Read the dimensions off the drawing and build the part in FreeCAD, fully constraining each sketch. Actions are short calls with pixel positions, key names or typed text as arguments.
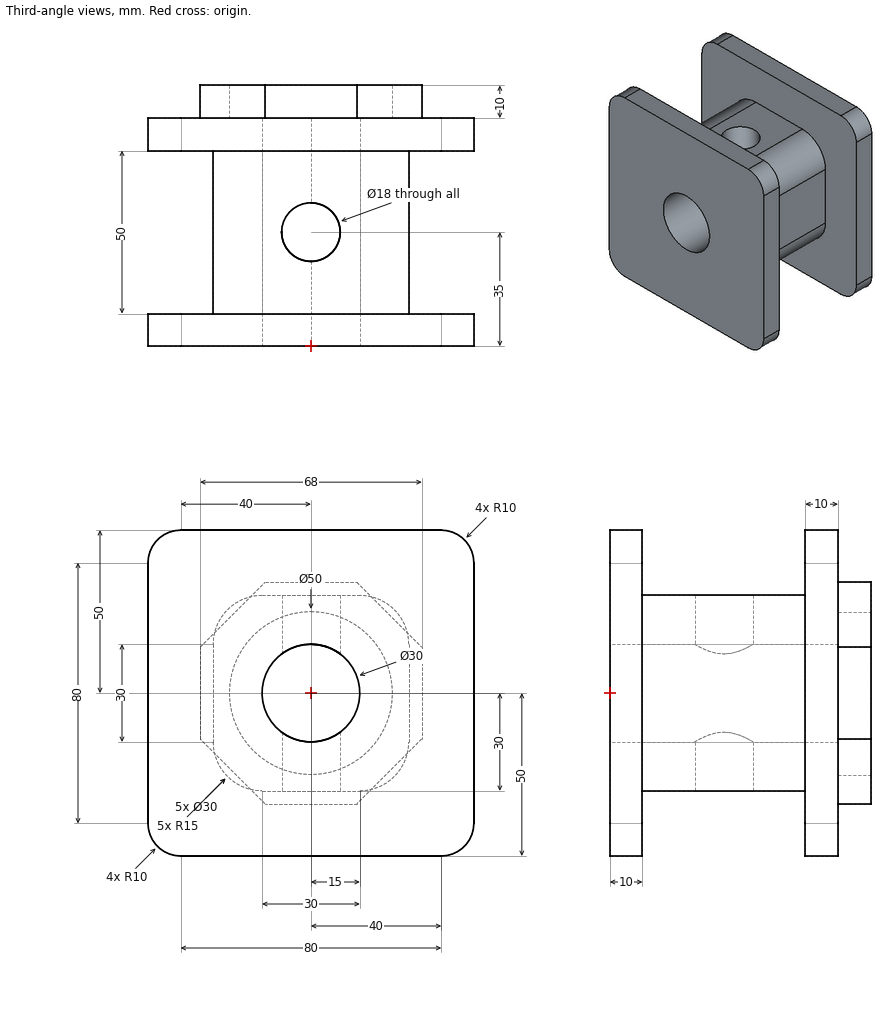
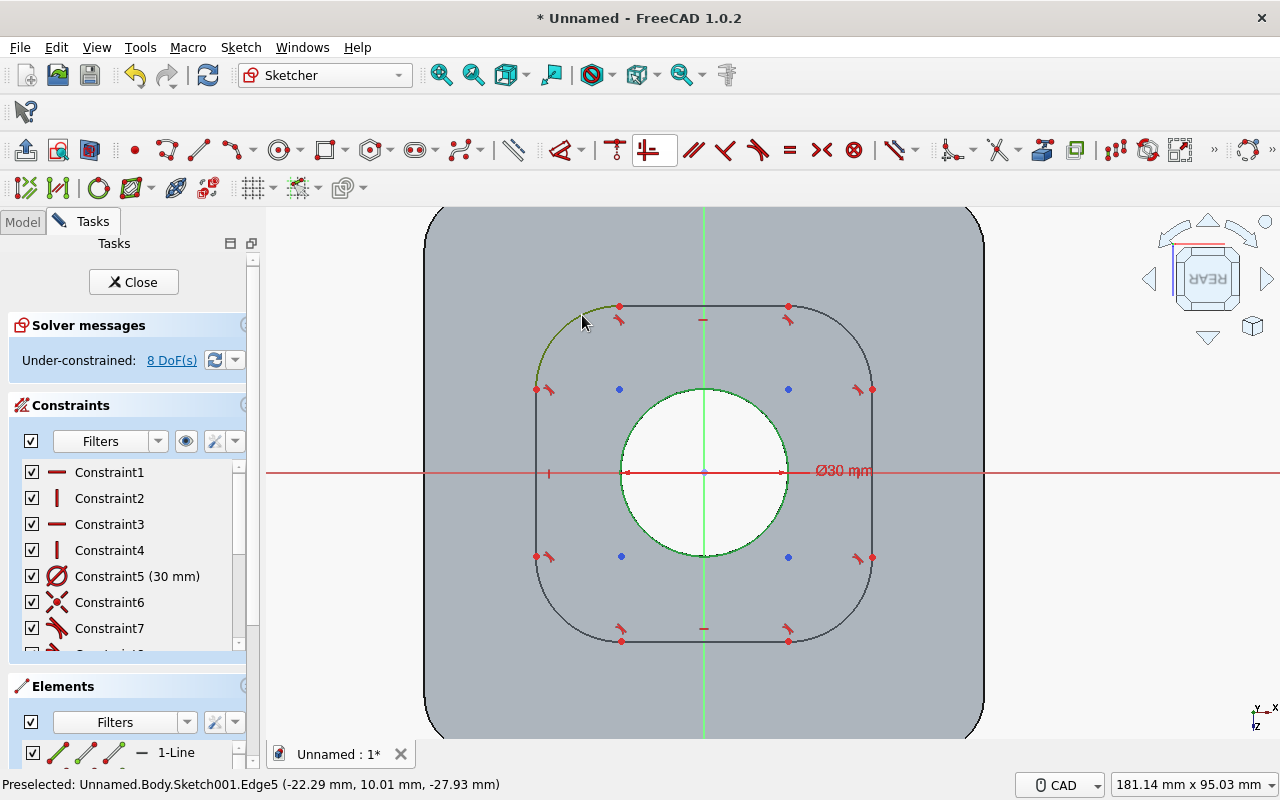
click(545, 595)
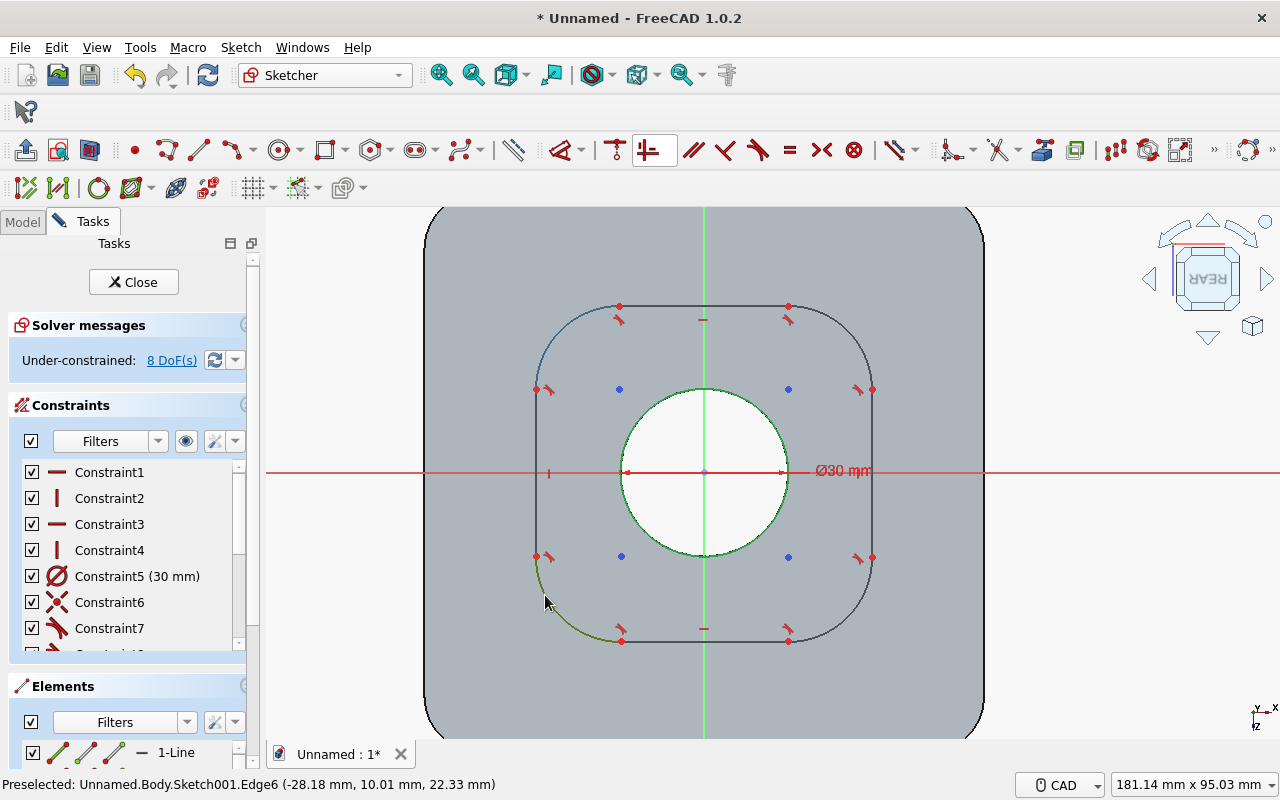
click(826, 633)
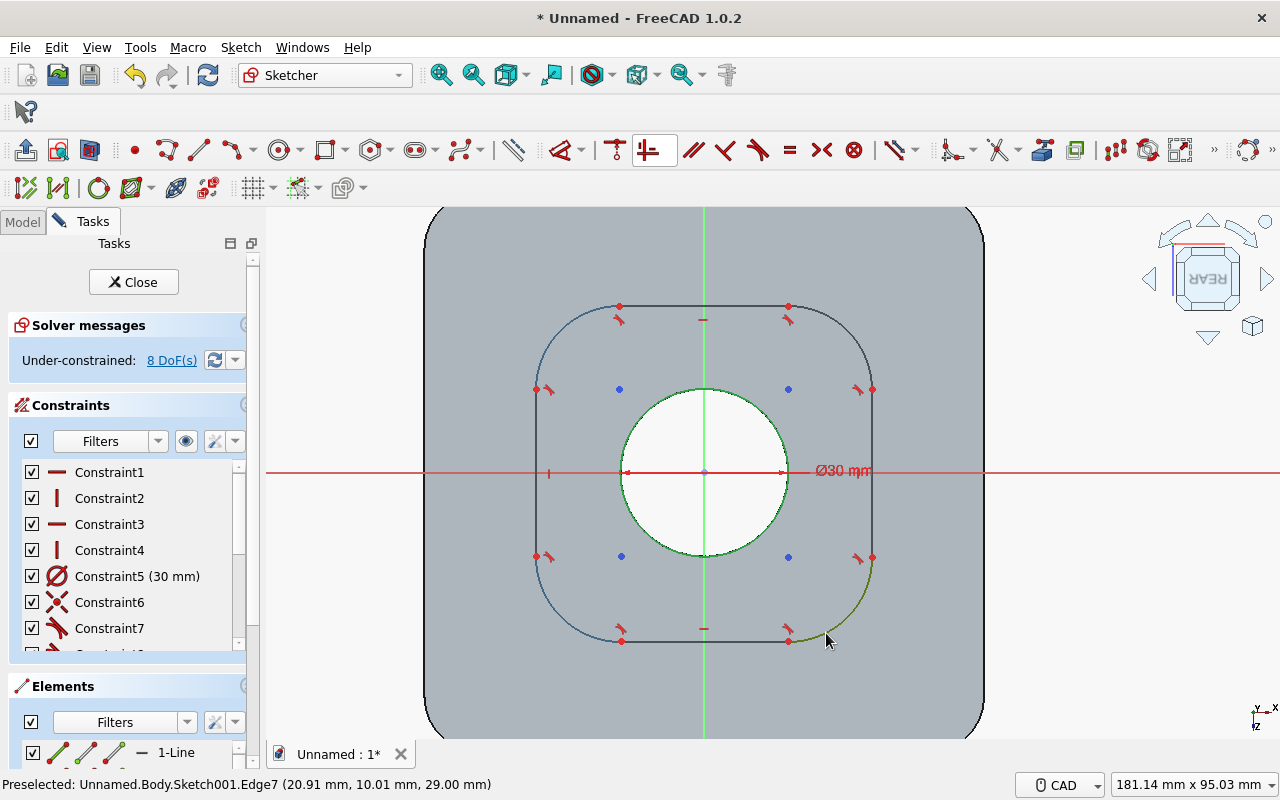
click(863, 352)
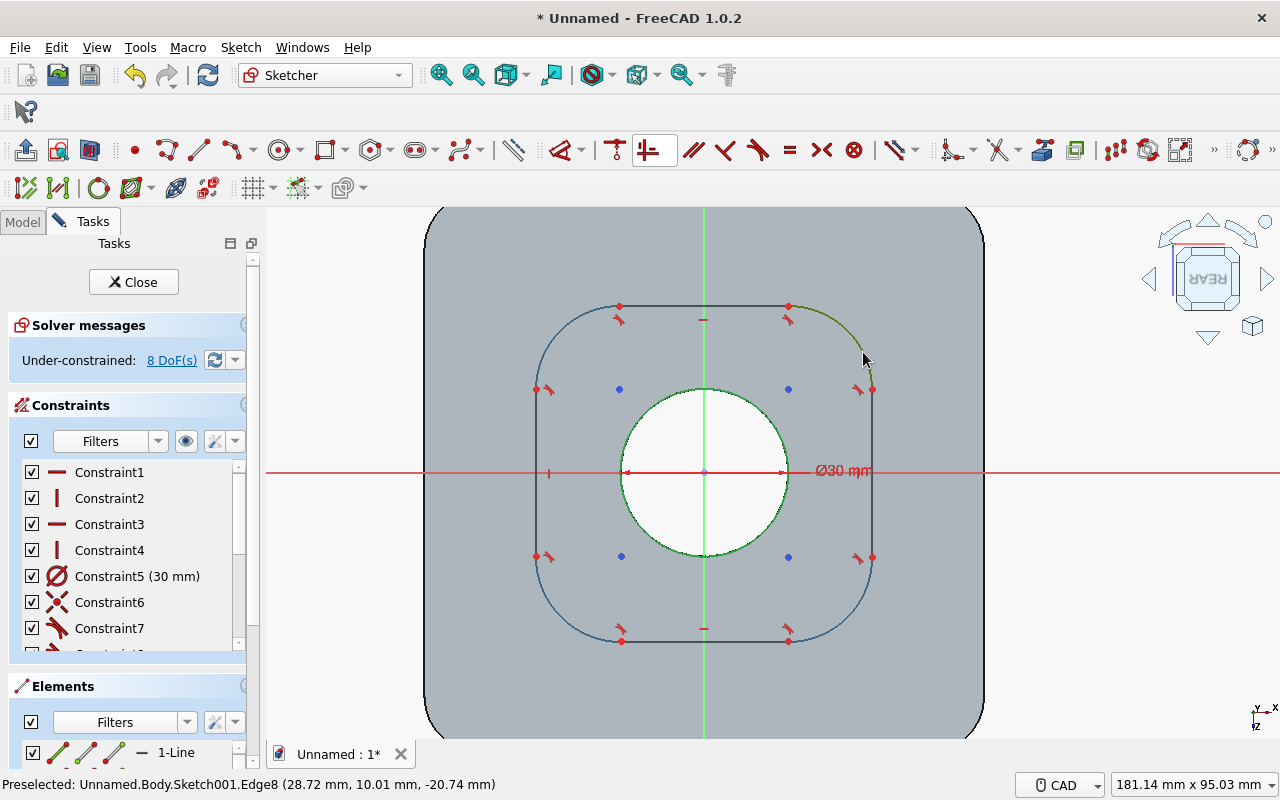
click(790, 150)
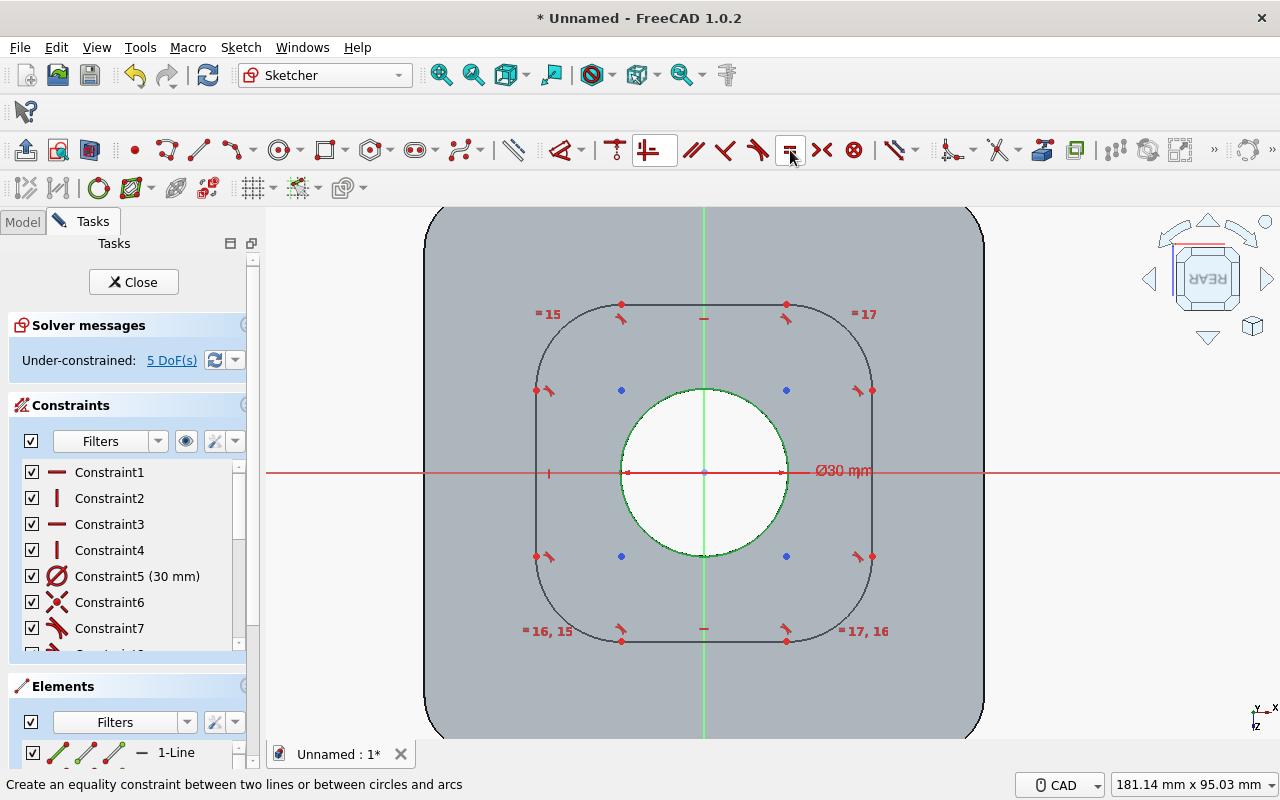
click(560, 150)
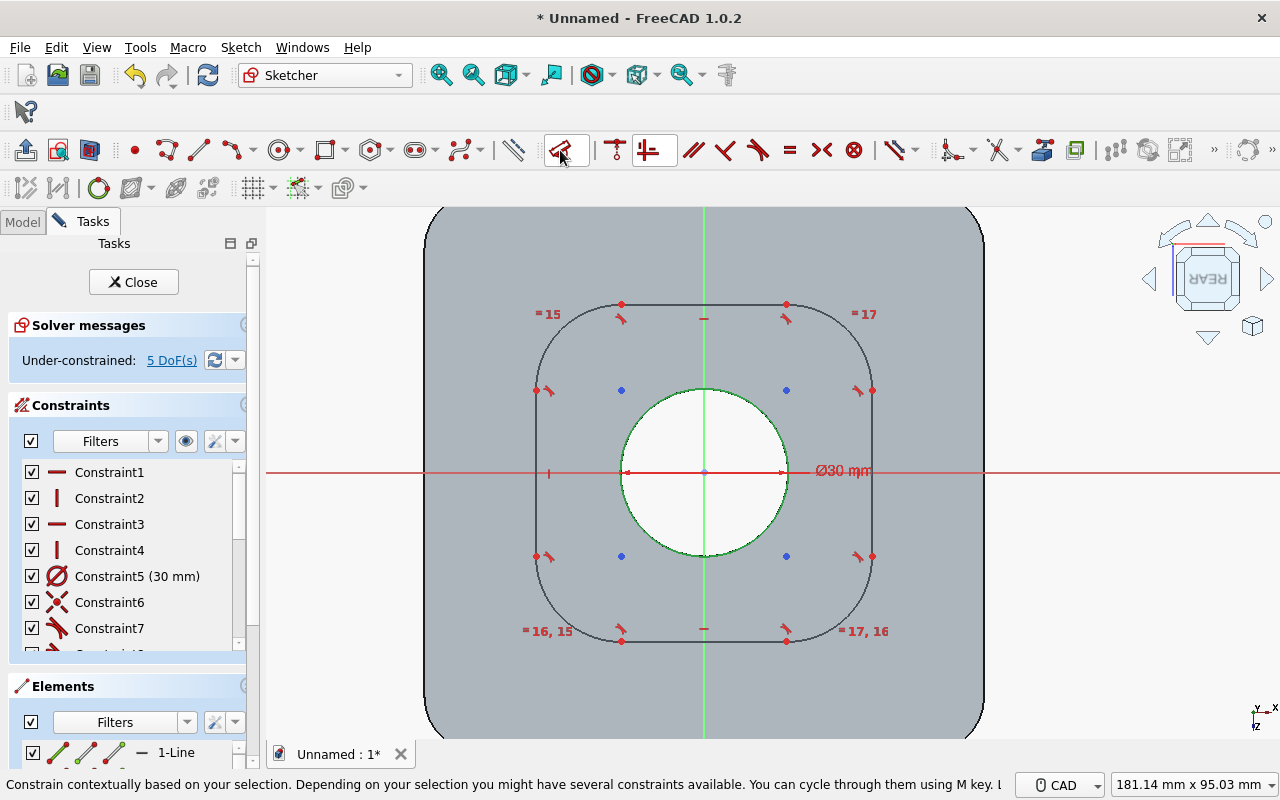
click(583, 314)
click(569, 285)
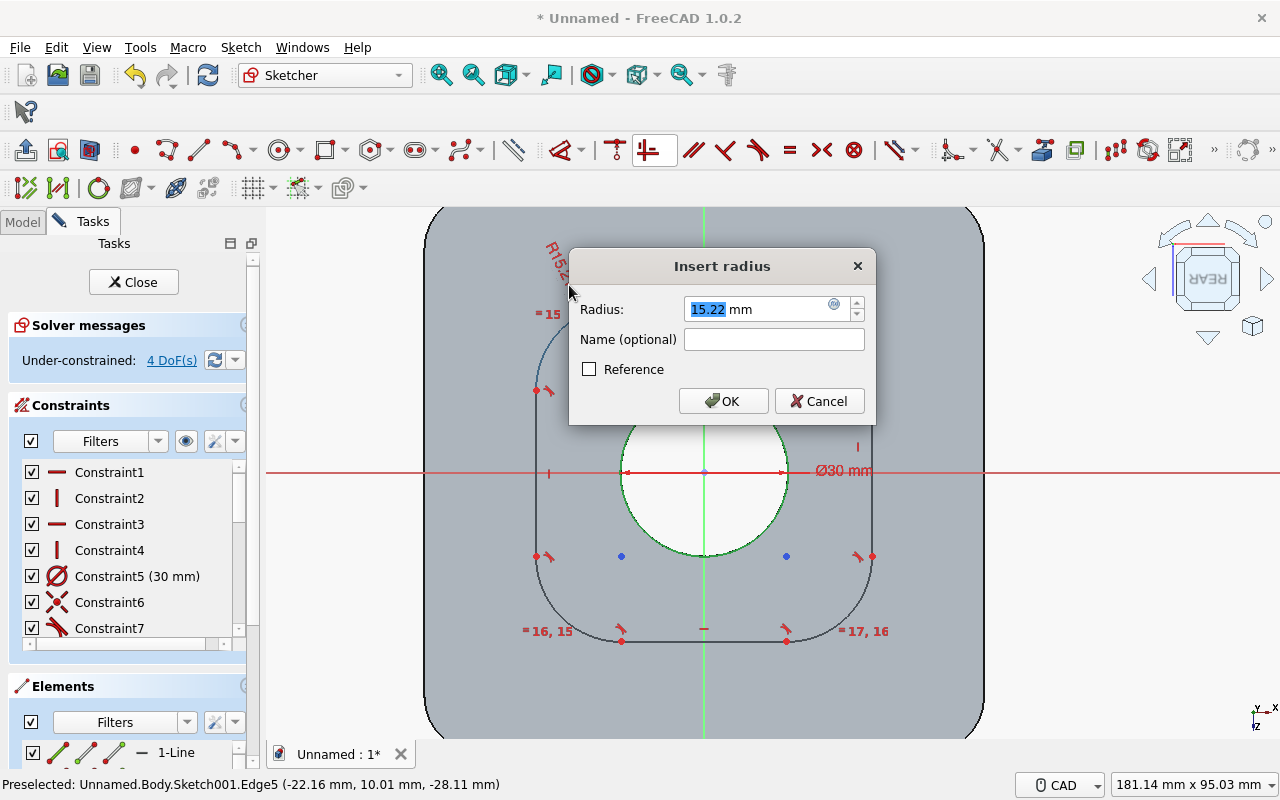
text(15)
key(Return)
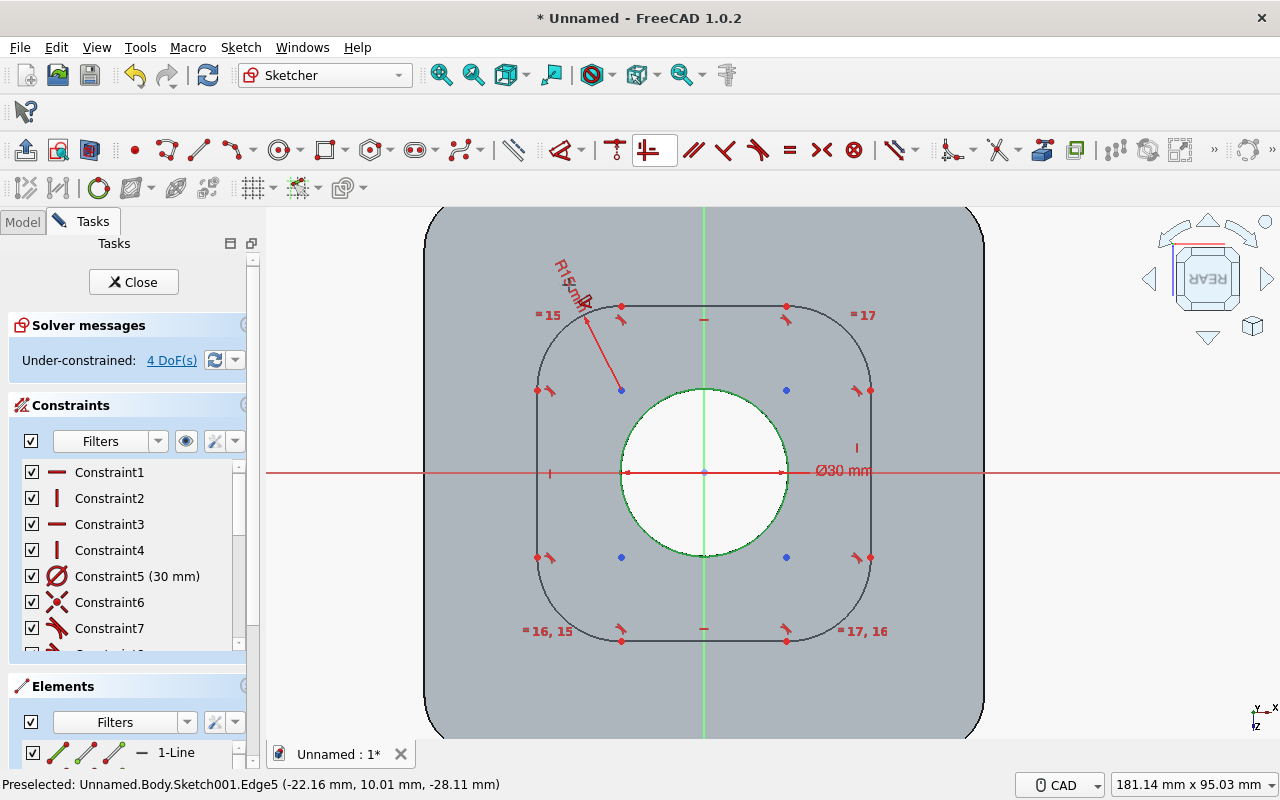
click(737, 306)
click(666, 272)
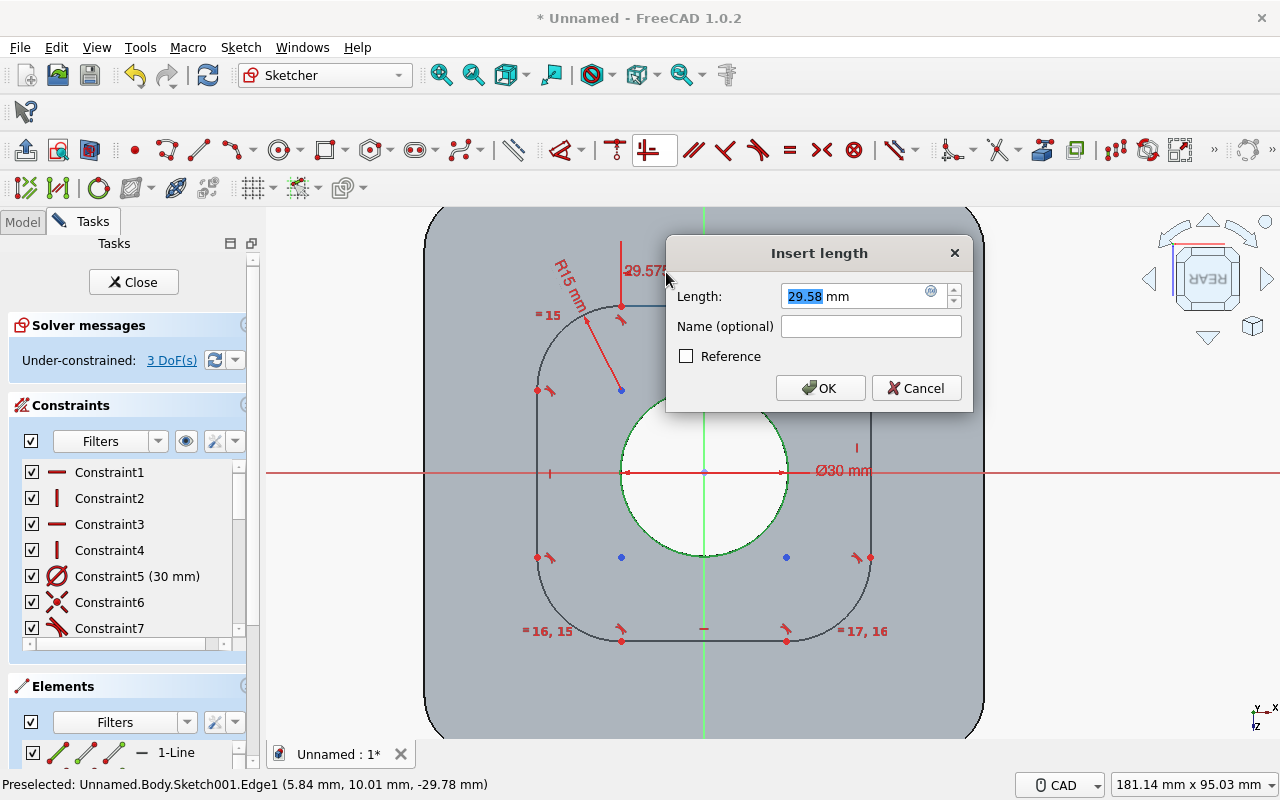
text(30)
key(Return)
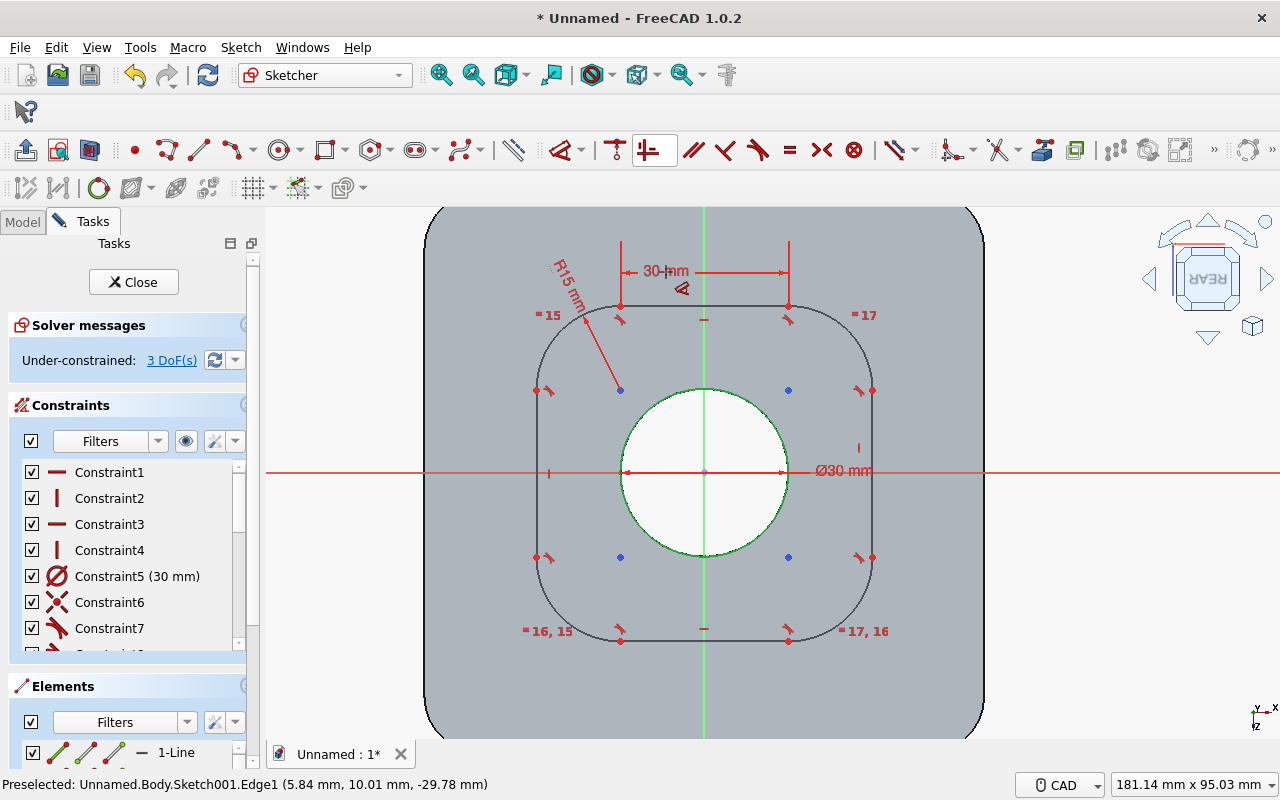
click(537, 440)
click(503, 435)